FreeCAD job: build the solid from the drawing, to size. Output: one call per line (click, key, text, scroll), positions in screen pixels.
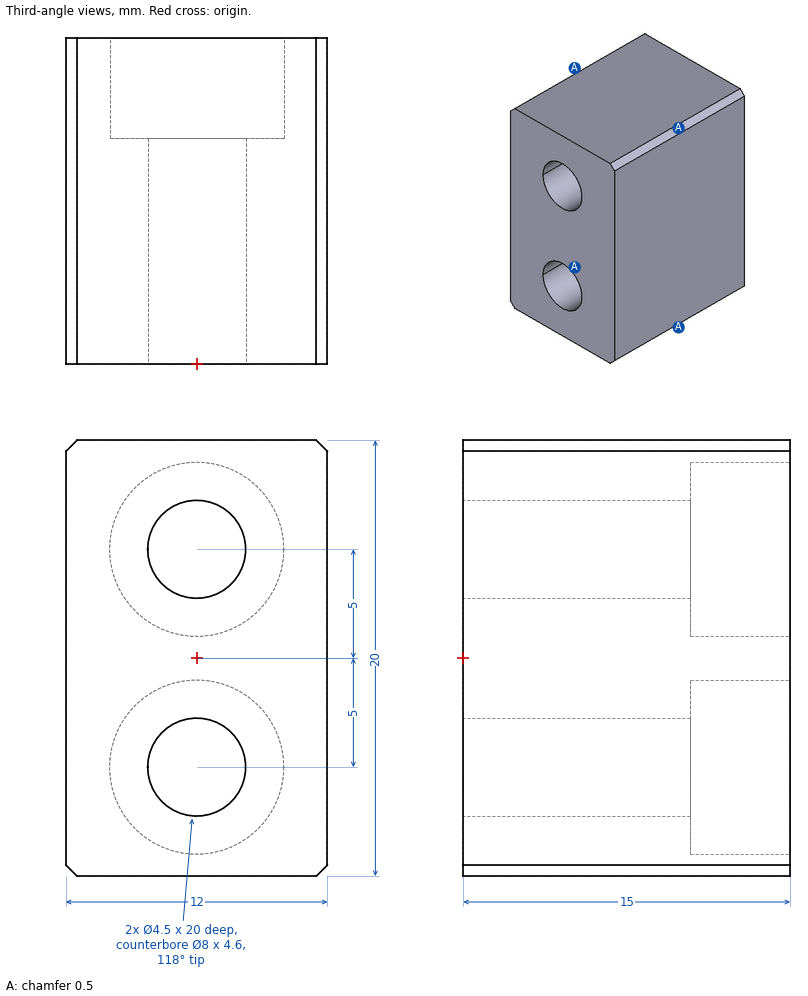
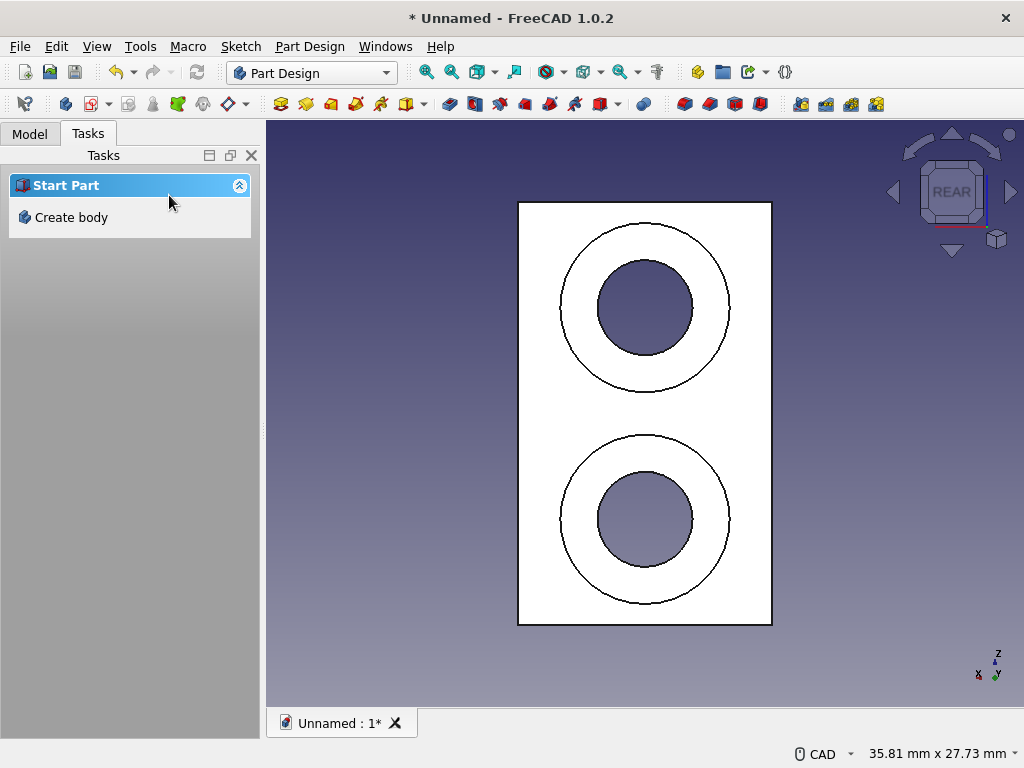
key(0)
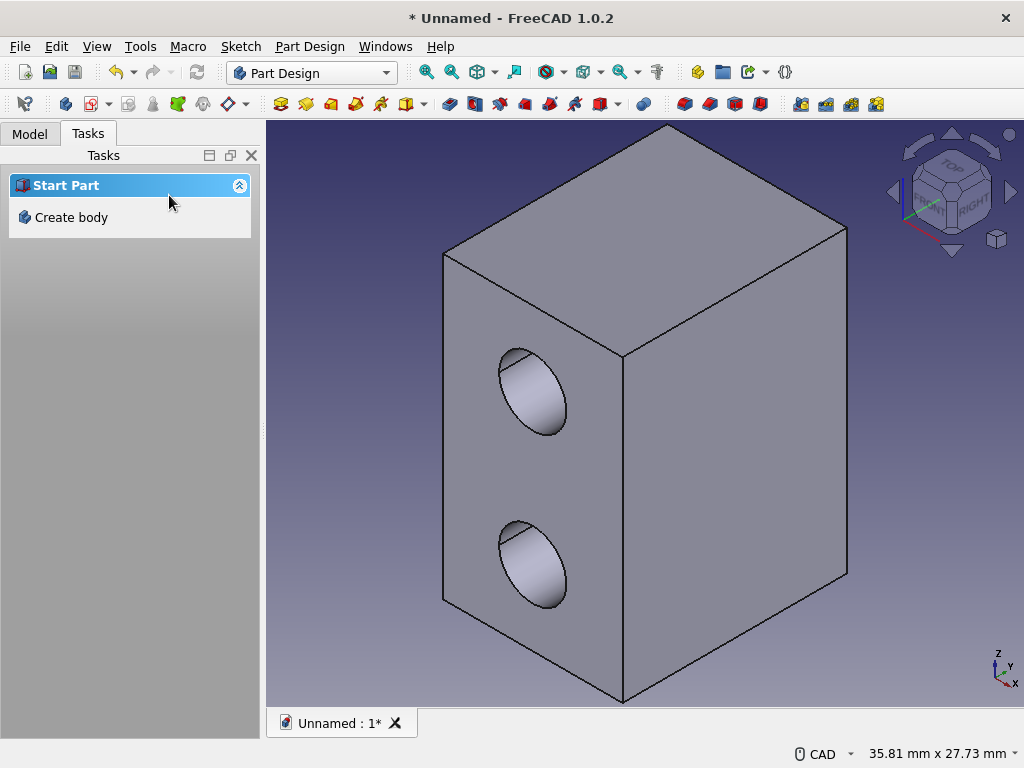
click(735, 292)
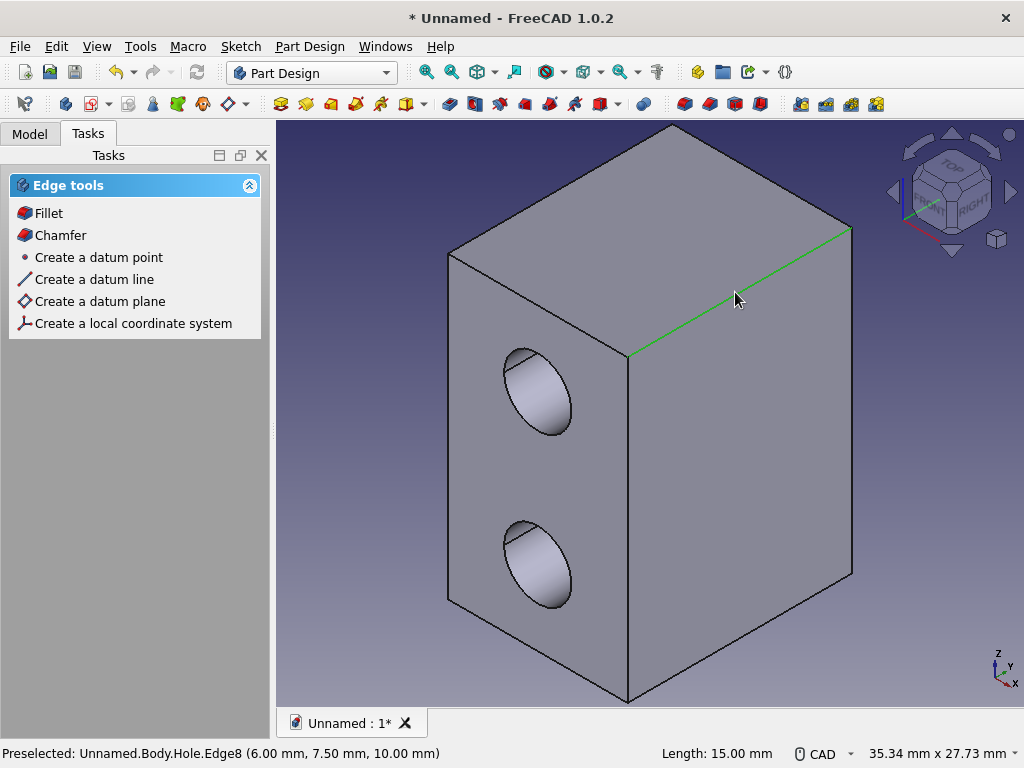
key(2)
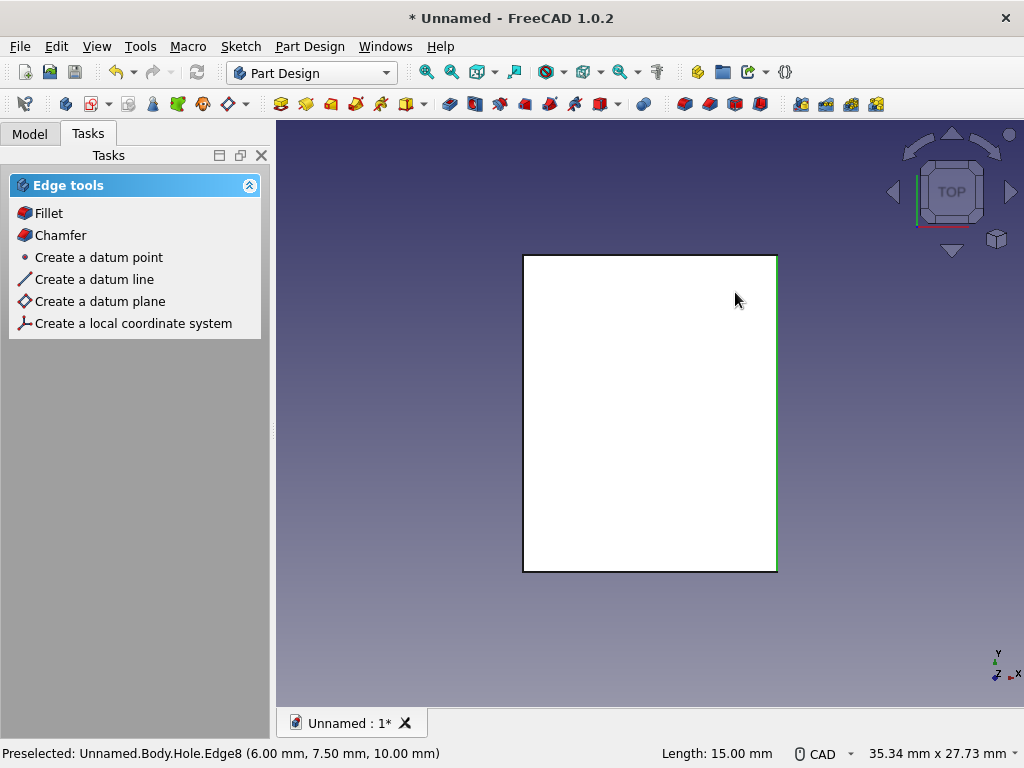
click(523, 412, ctrl)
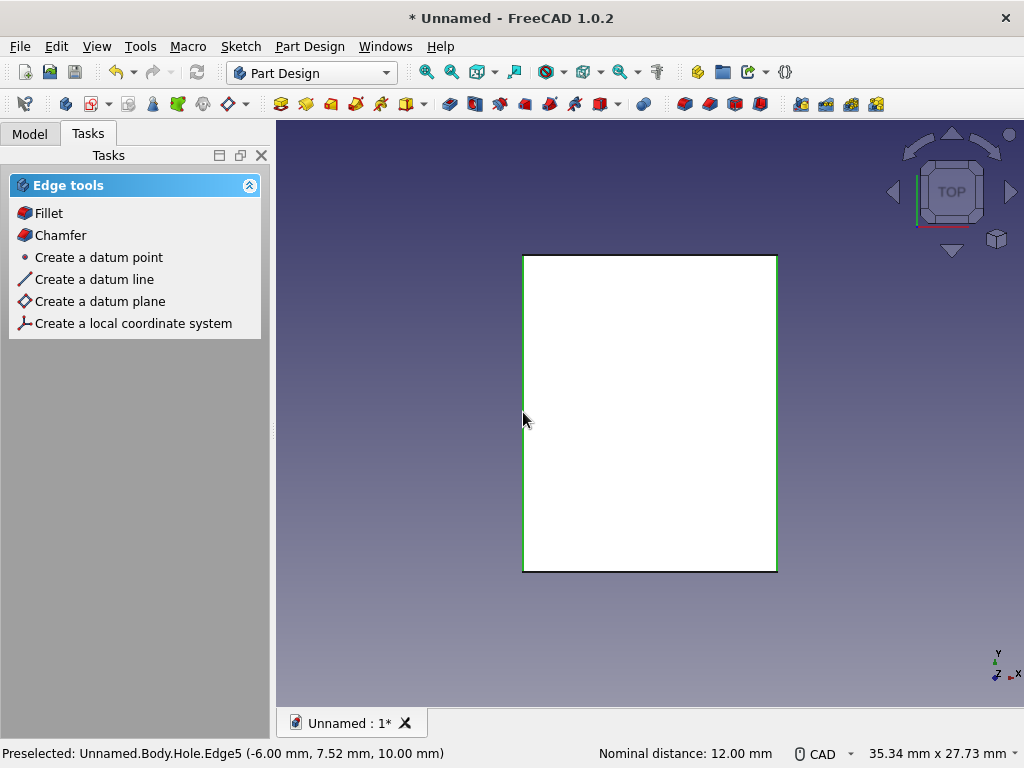
key(1)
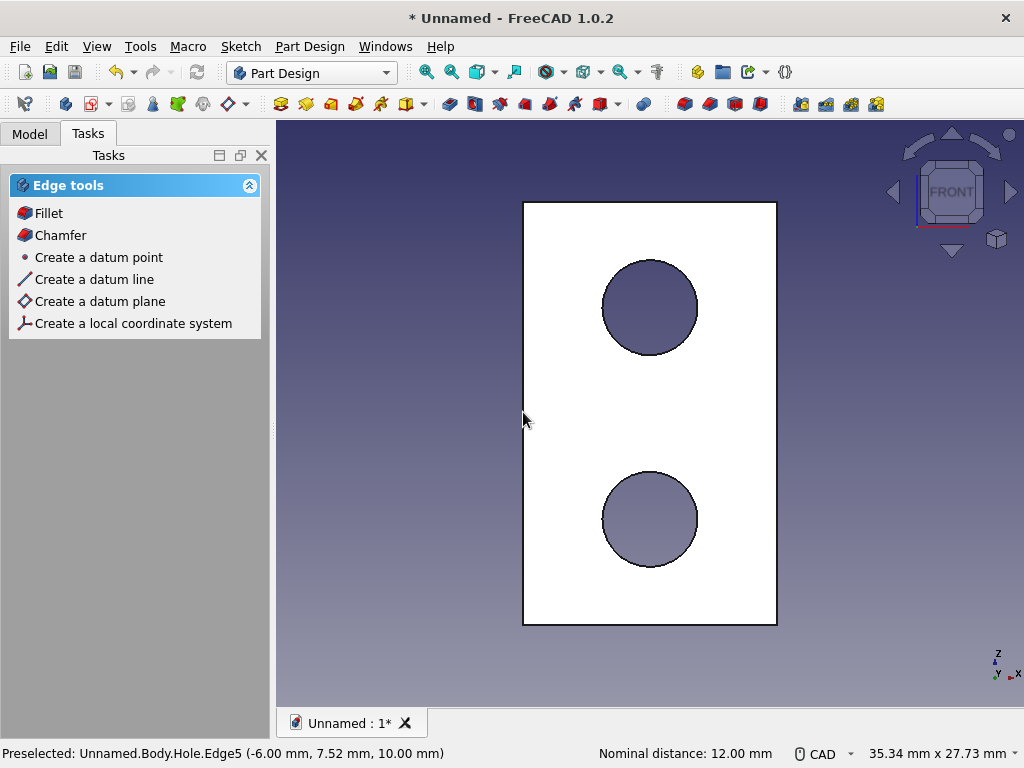
key(3)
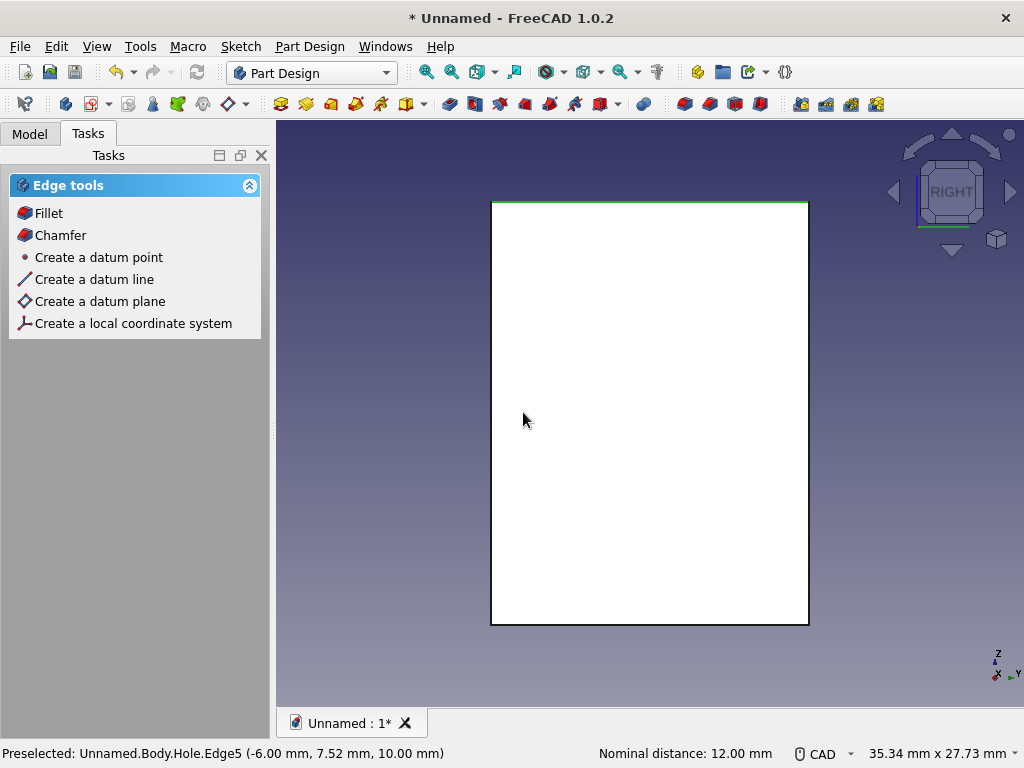
click(650, 624, ctrl)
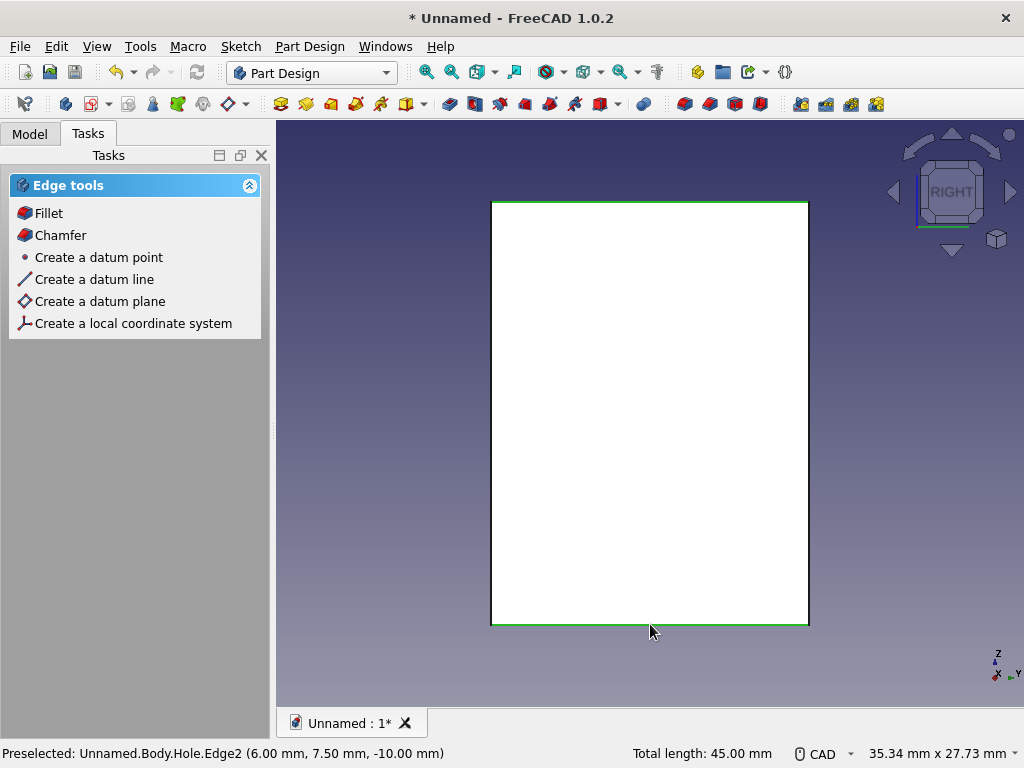
key(5)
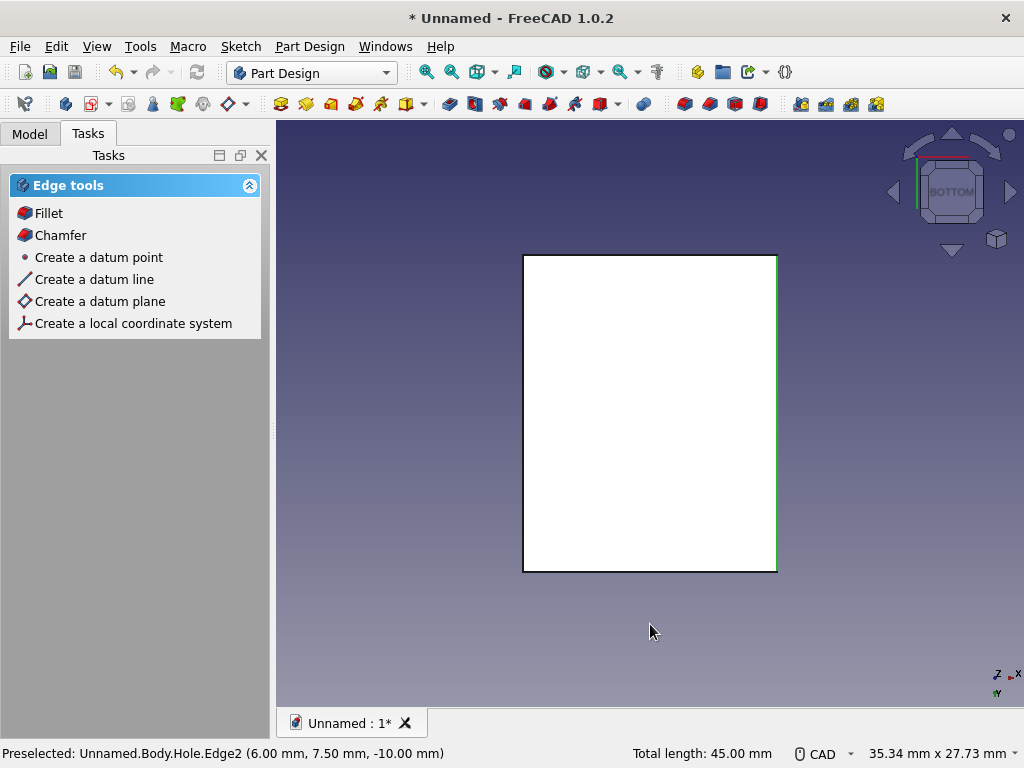
click(523, 413, ctrl)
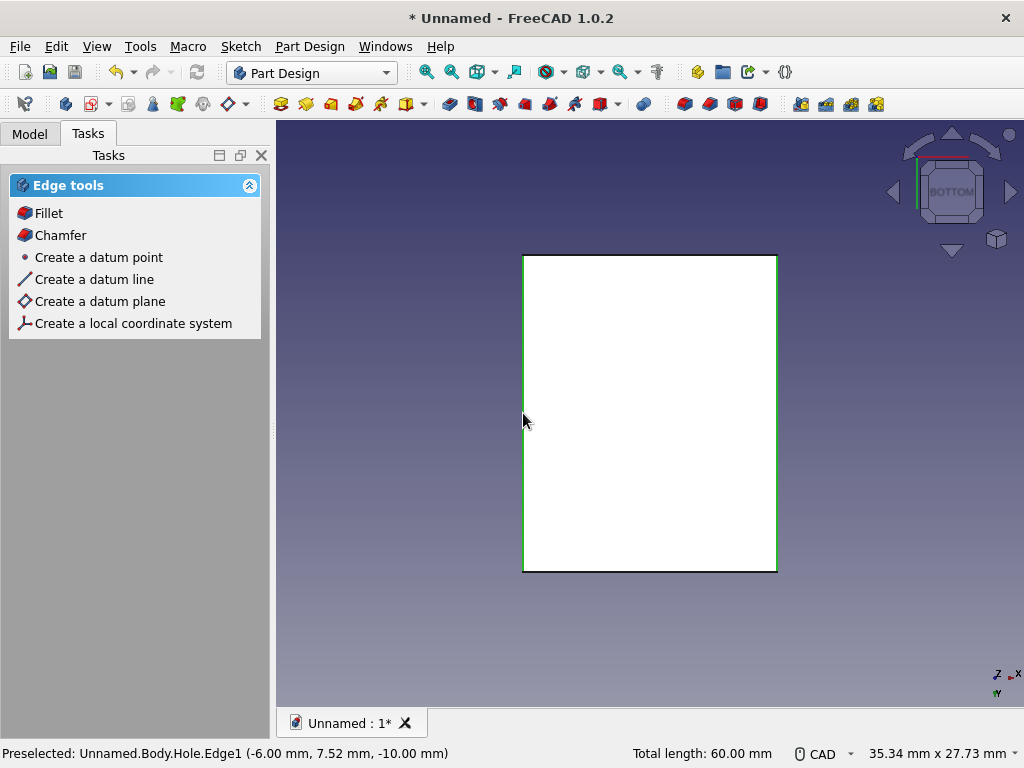
click(710, 104)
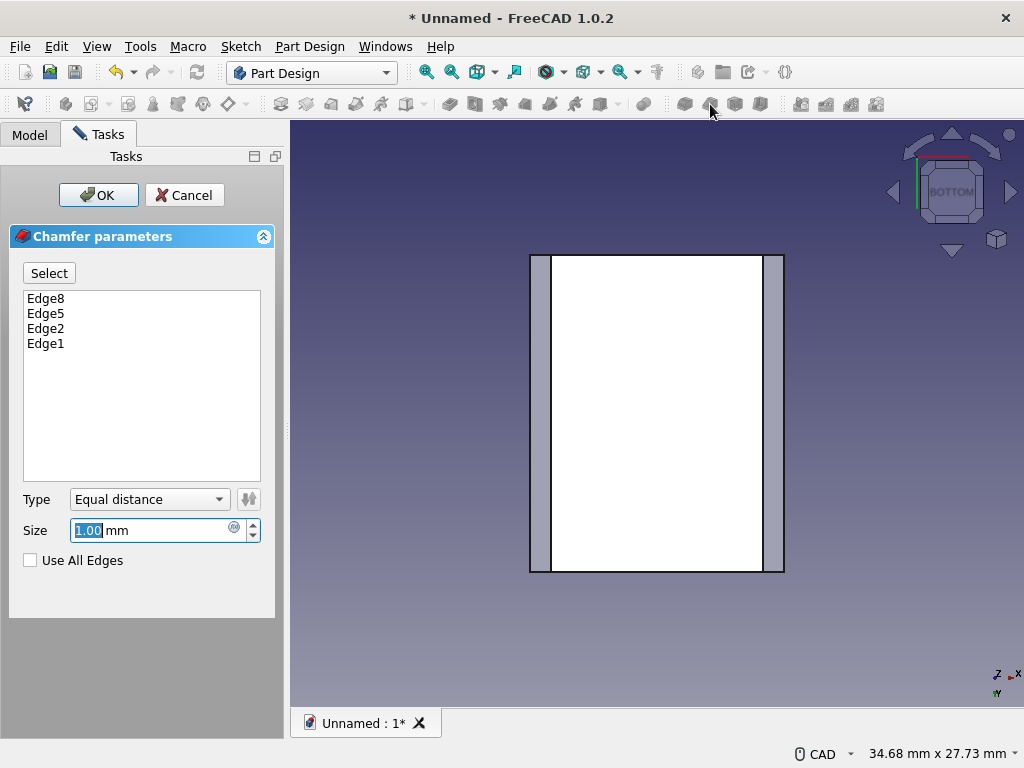
text(0.5)
key(Tab)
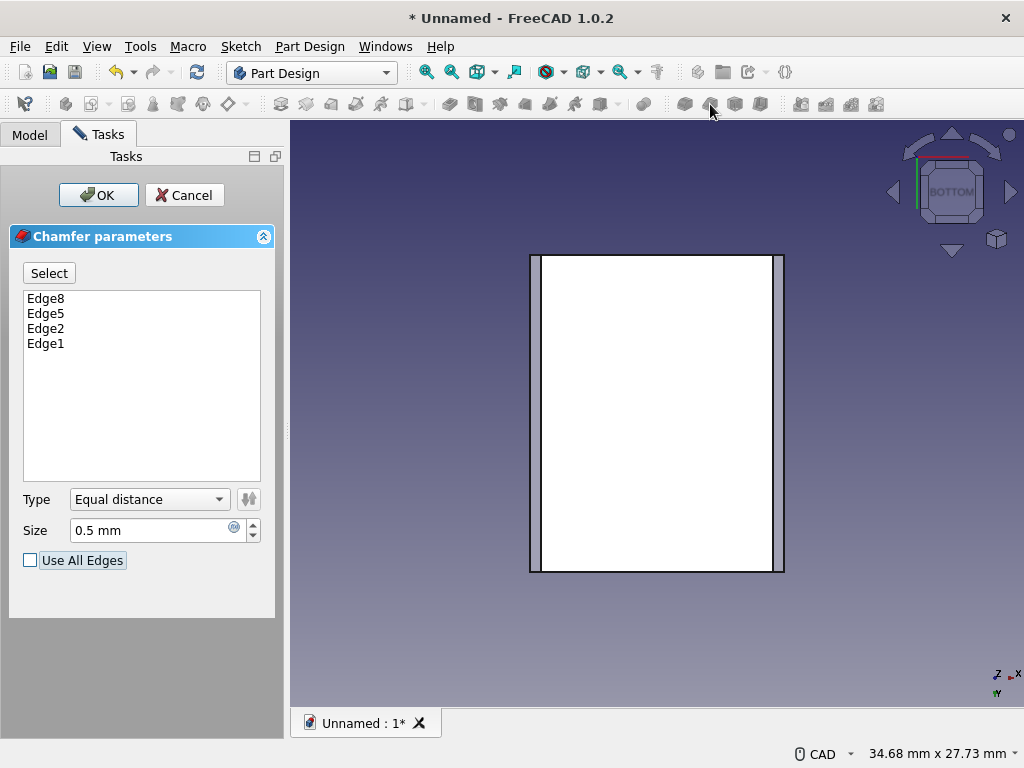
click(99, 195)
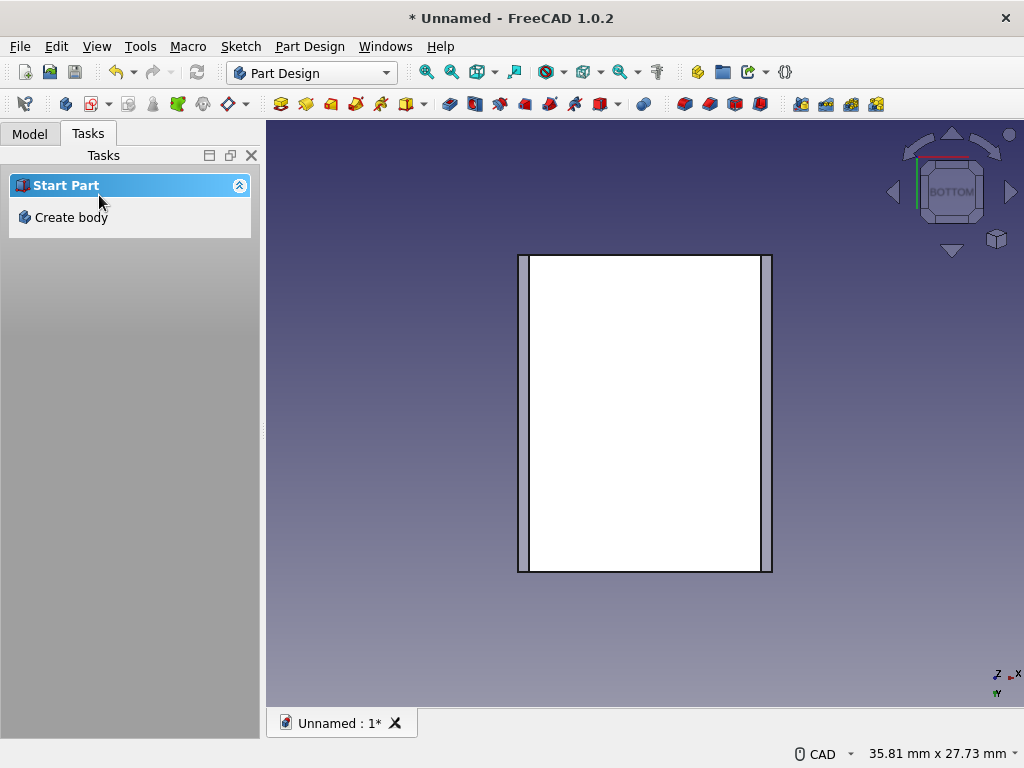
key(0)